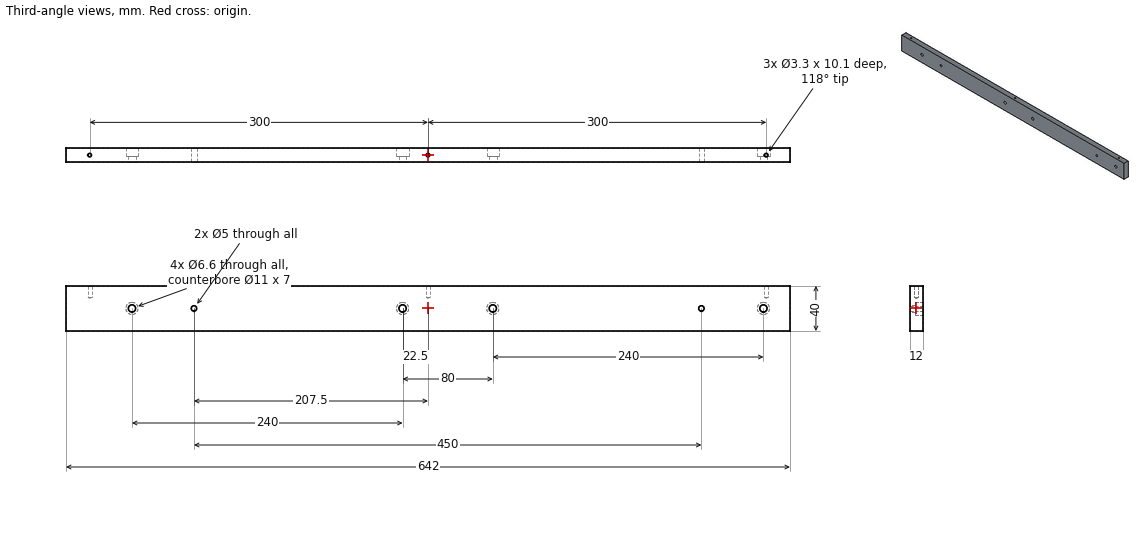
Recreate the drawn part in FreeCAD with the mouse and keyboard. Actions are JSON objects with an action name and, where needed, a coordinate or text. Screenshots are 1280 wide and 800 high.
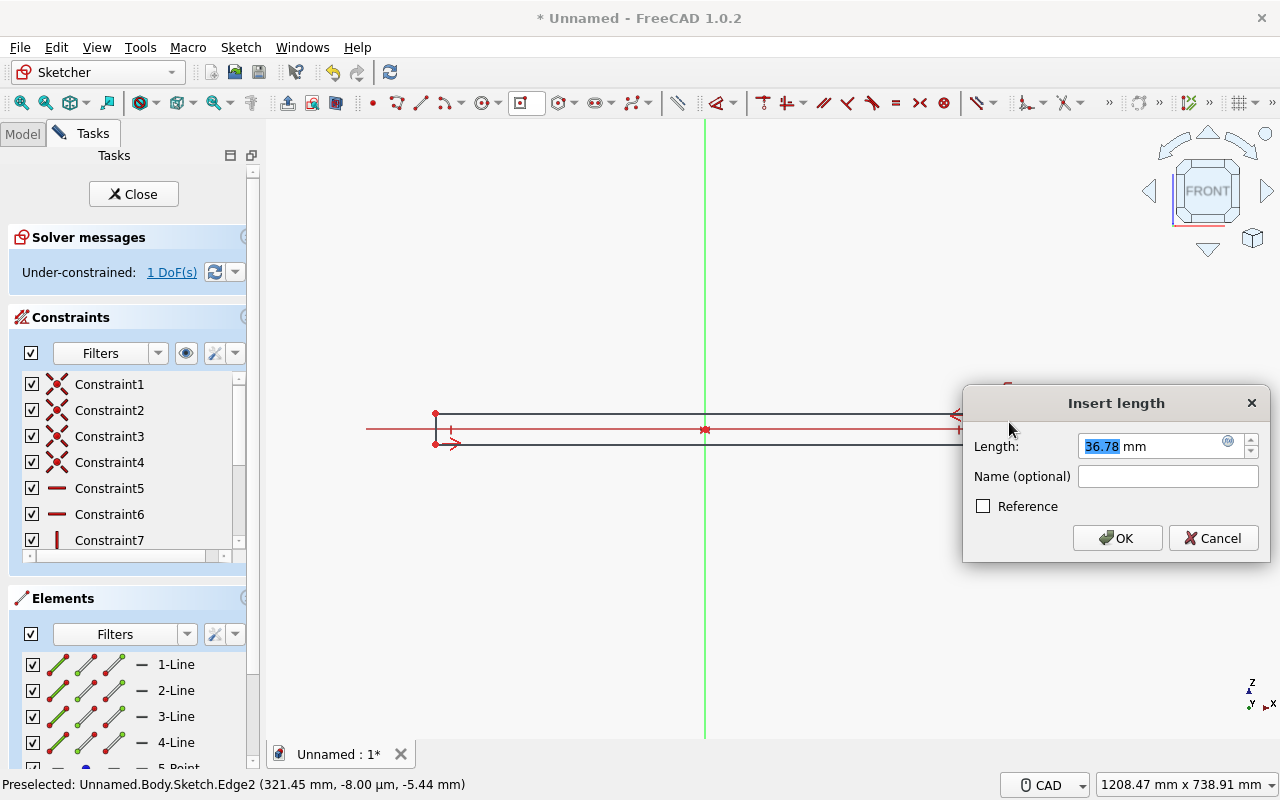
{"action": "type", "text": "40"}
{"action": "key", "text": "Return"}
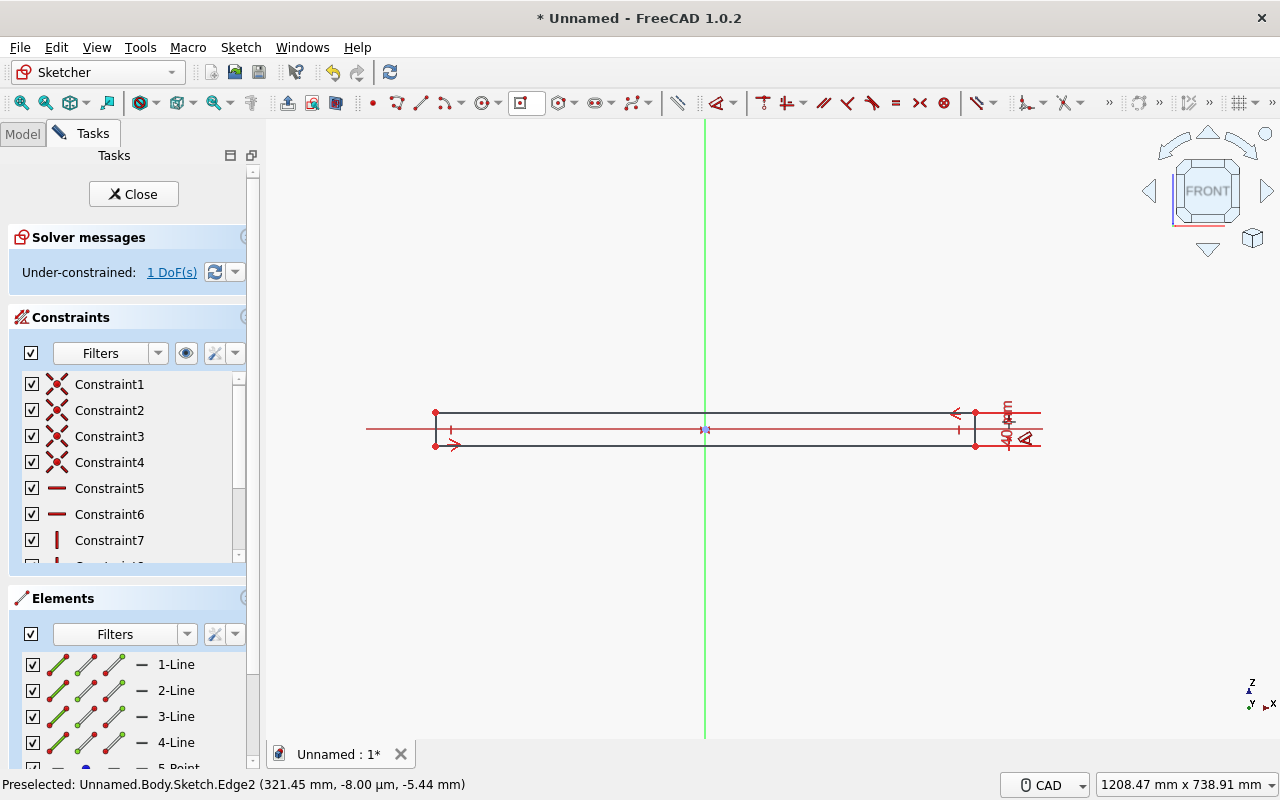
{"action": "left_click", "coordinate": [597, 446]}
{"action": "left_click", "coordinate": [581, 480]}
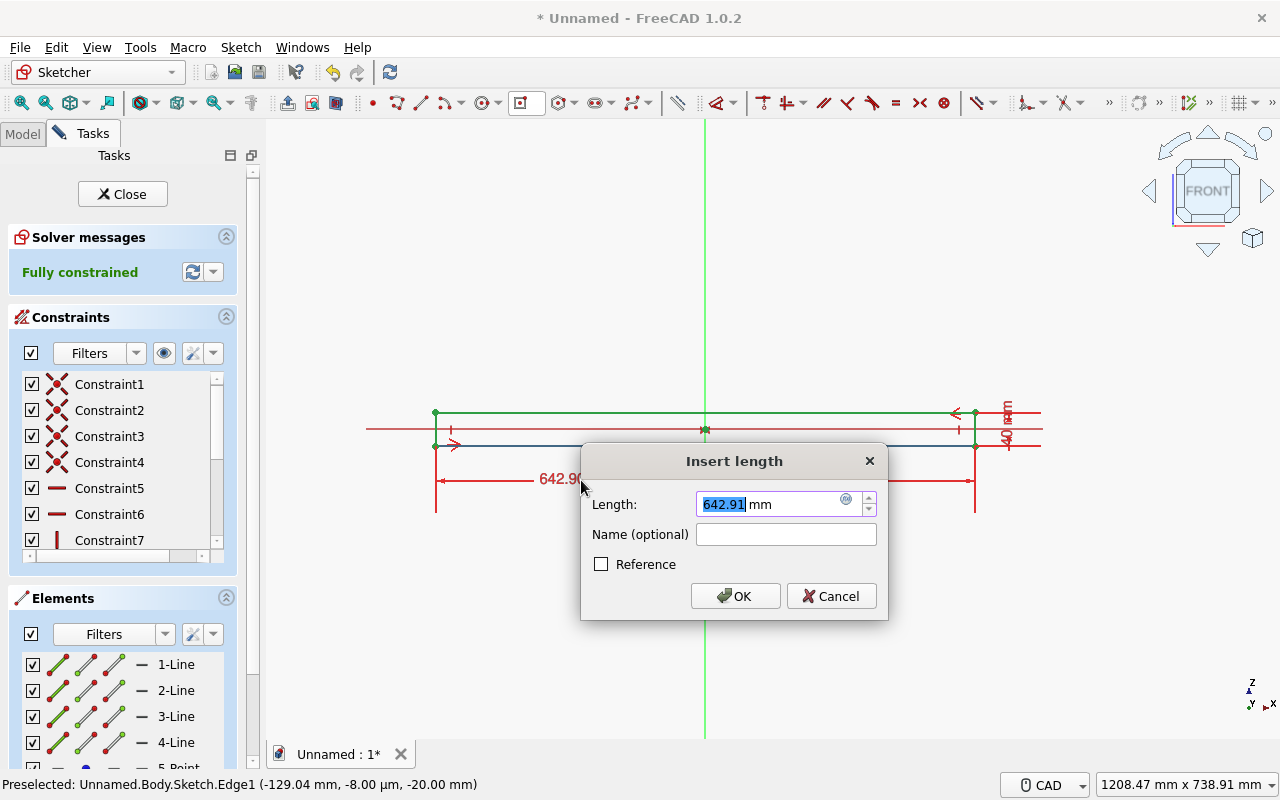
{"action": "type", "text": "642"}
{"action": "key", "text": "Return"}
{"action": "key", "text": "Escape"}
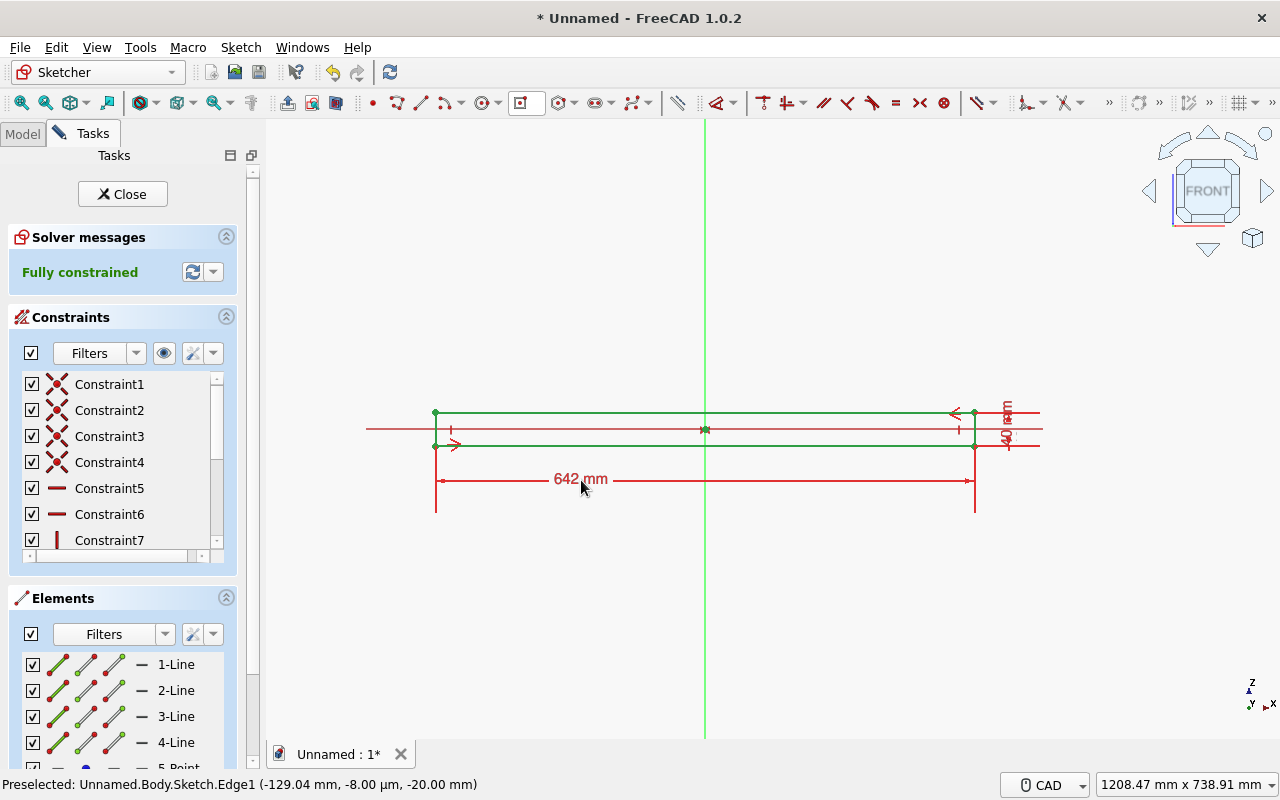
{"action": "left_click", "coordinate": [123, 194]}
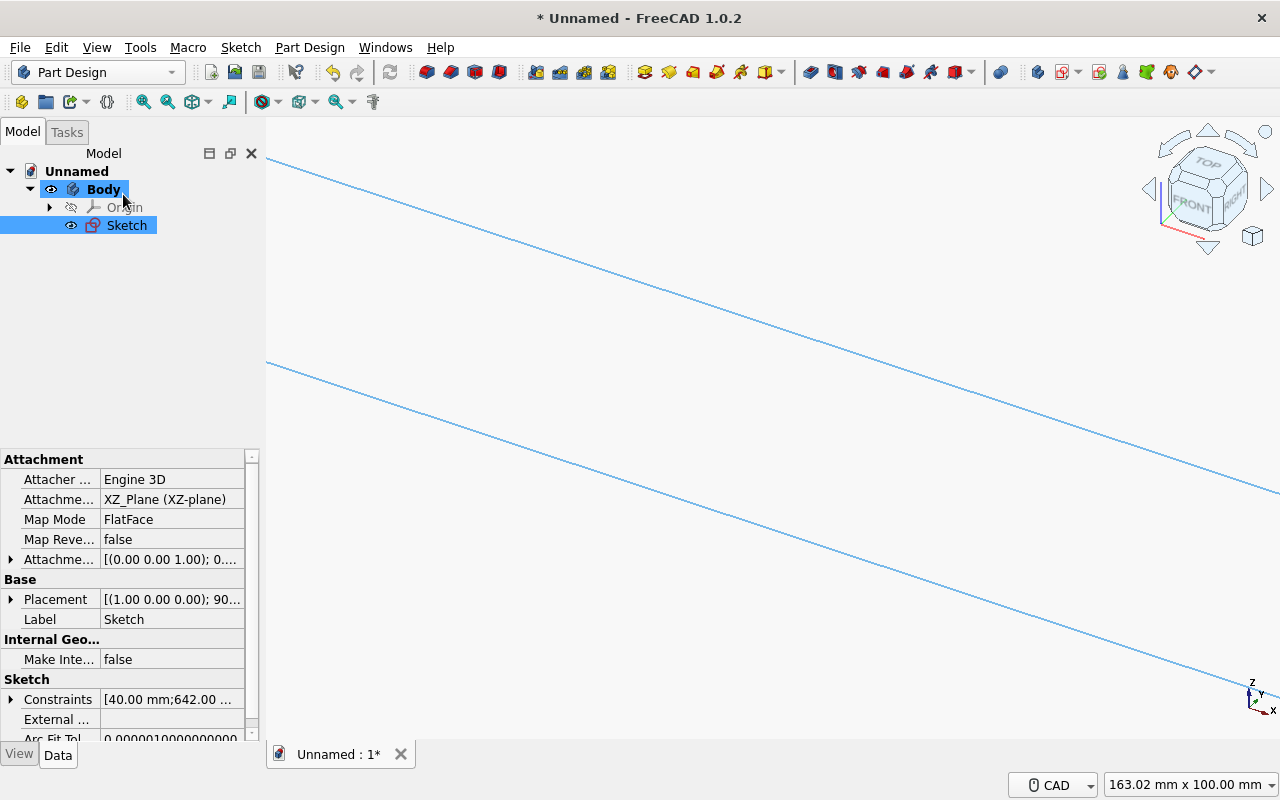
{"action": "left_click", "coordinate": [646, 72]}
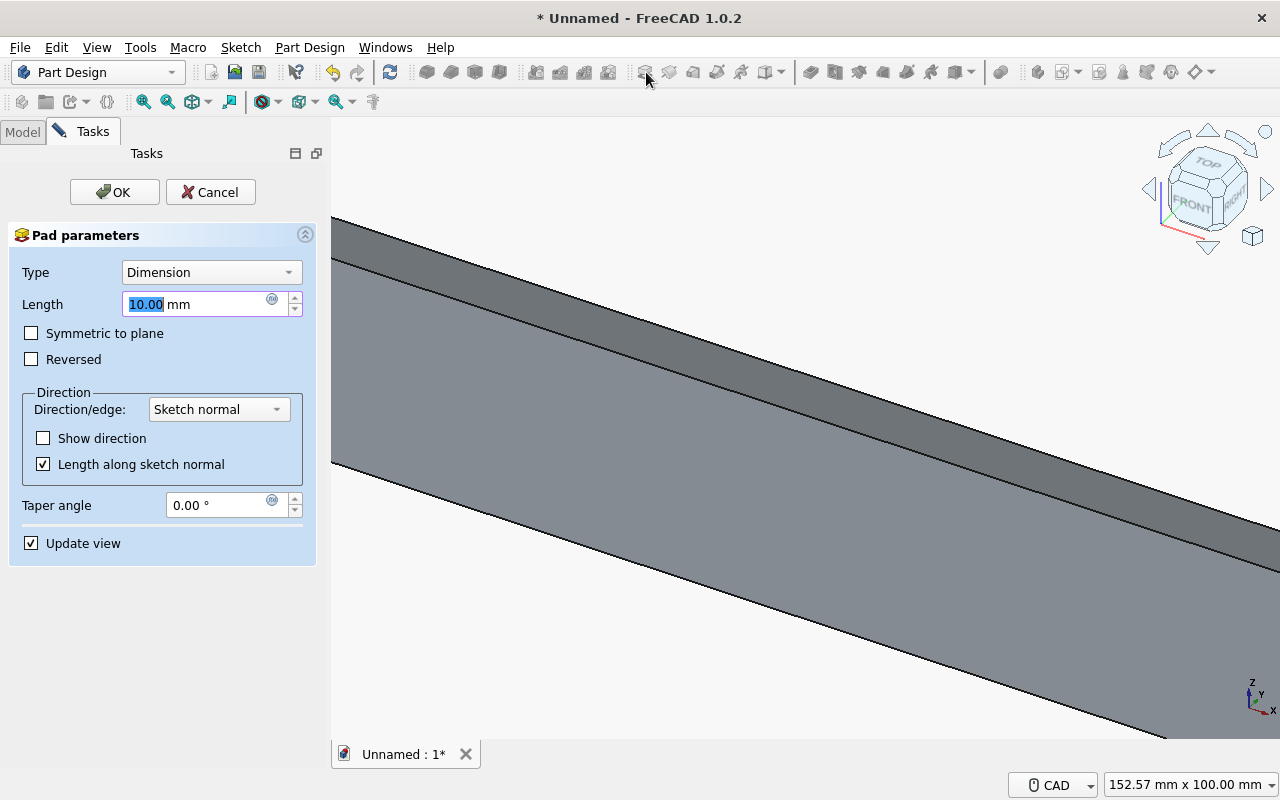
{"action": "type", "text": "12"}
{"action": "key", "text": "Tab"}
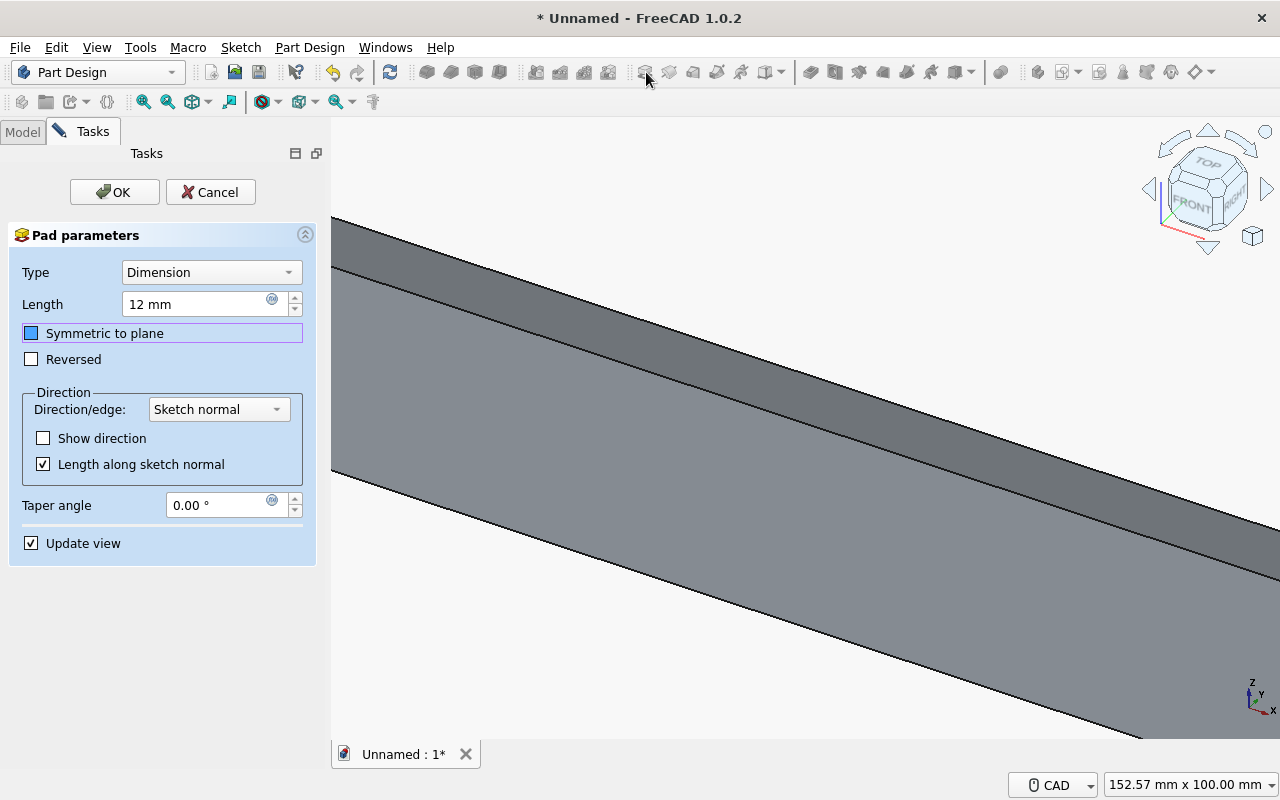
{"action": "left_click", "coordinate": [30, 333]}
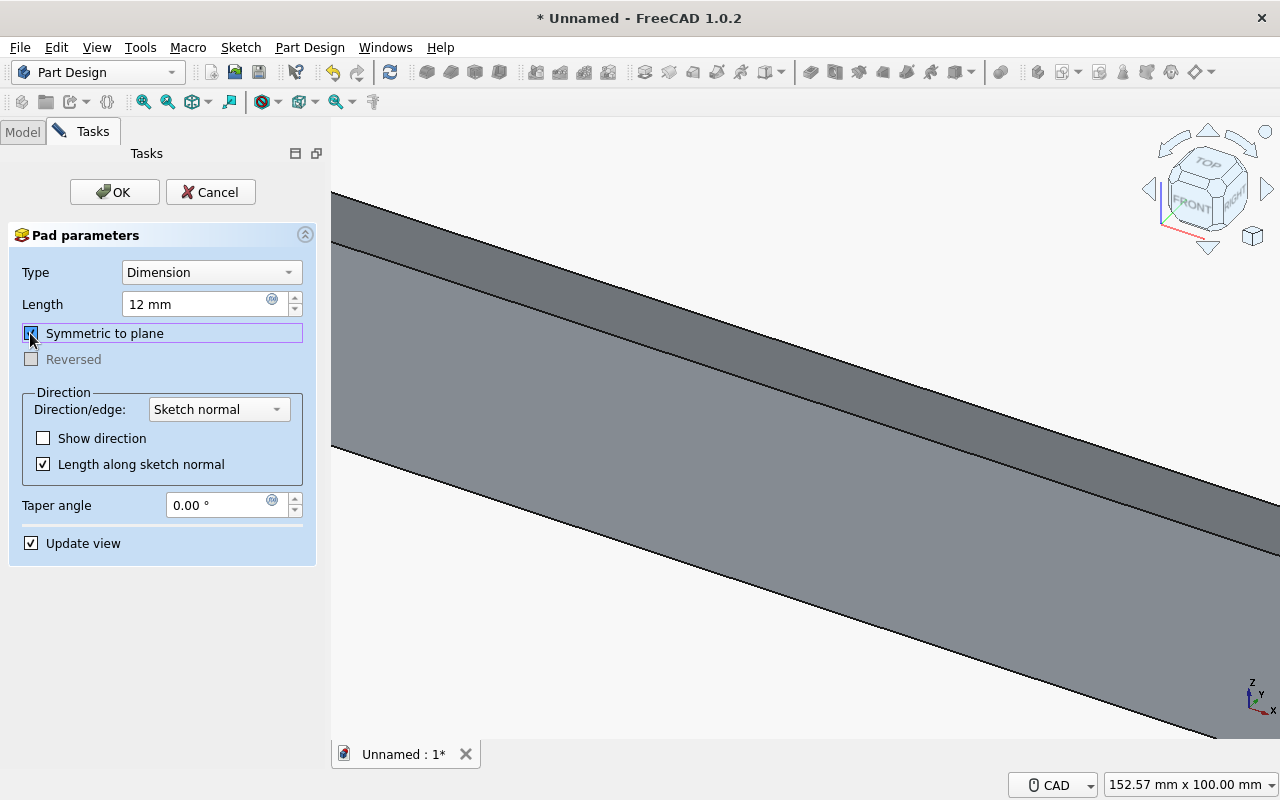
{"action": "left_click", "coordinate": [115, 192]}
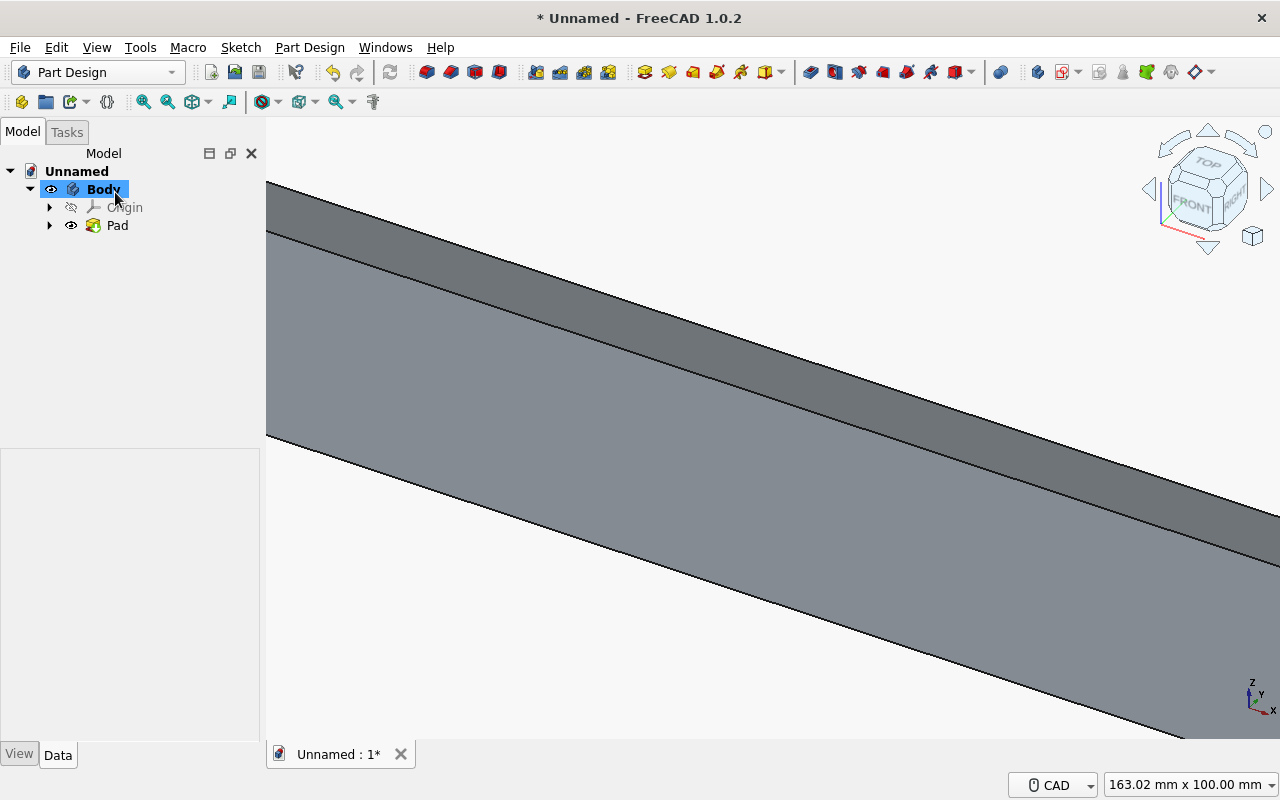
{"action": "left_click", "coordinate": [144, 102]}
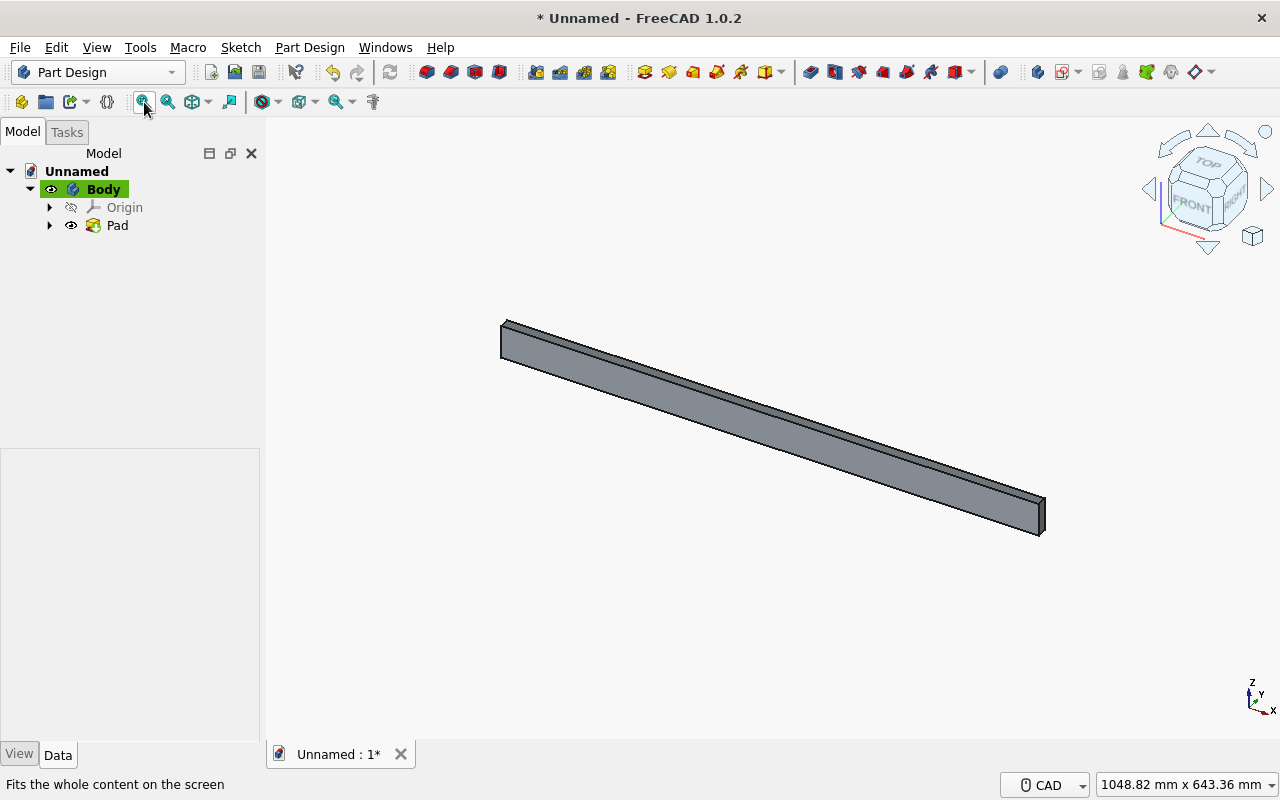
{"action": "key", "text": "4"}